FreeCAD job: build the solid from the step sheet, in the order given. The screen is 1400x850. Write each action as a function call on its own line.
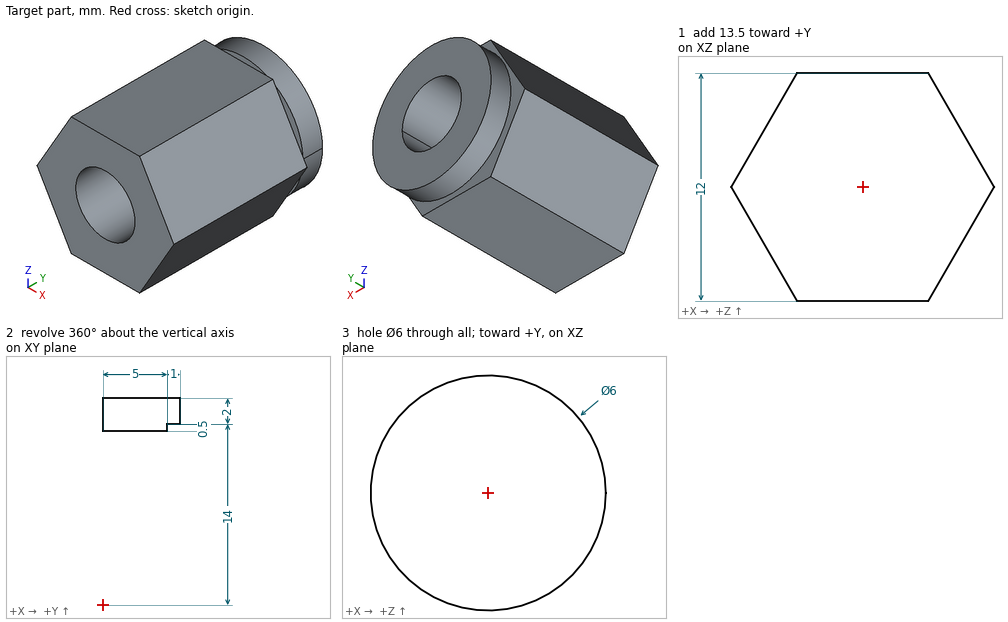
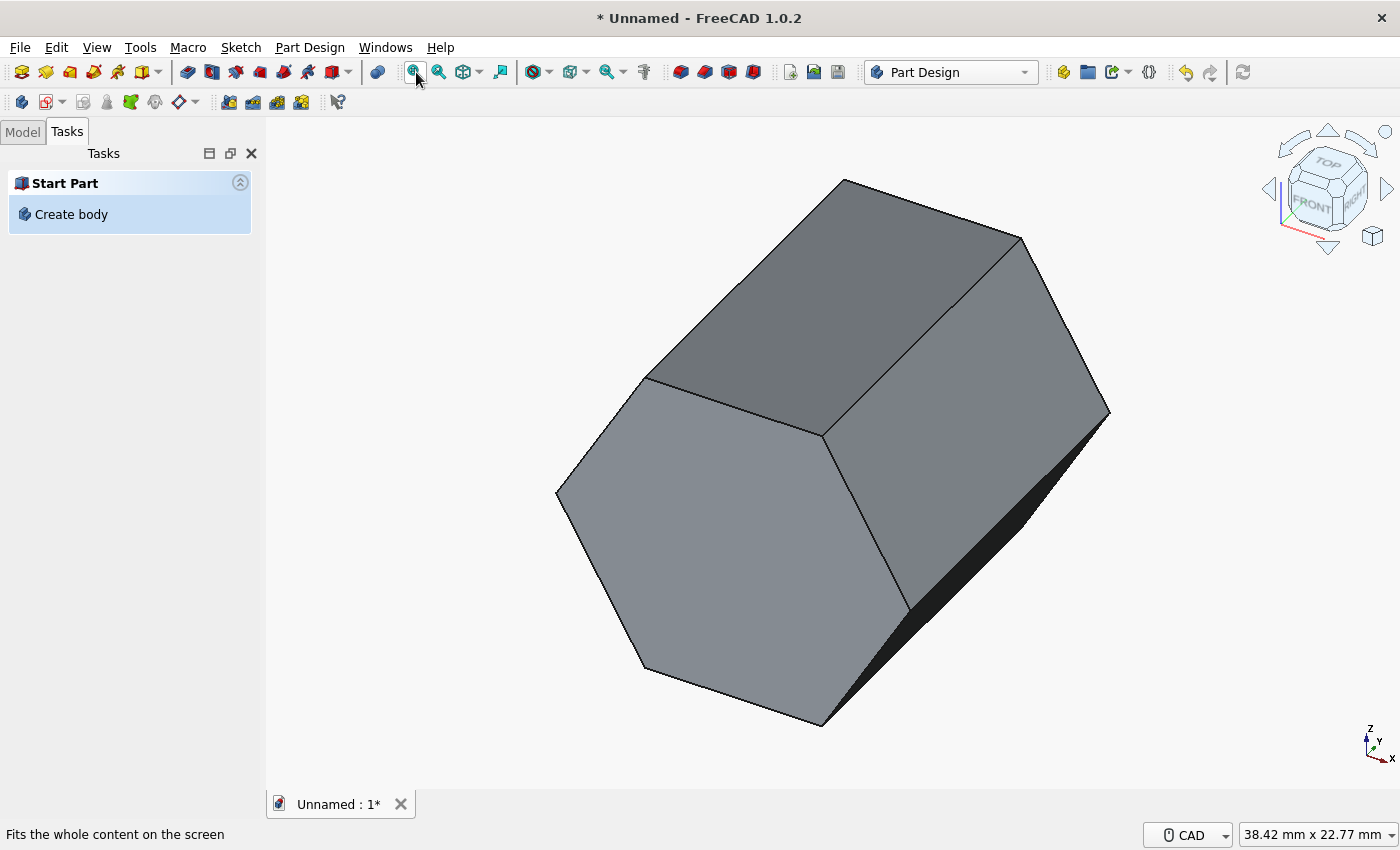
click(46, 102)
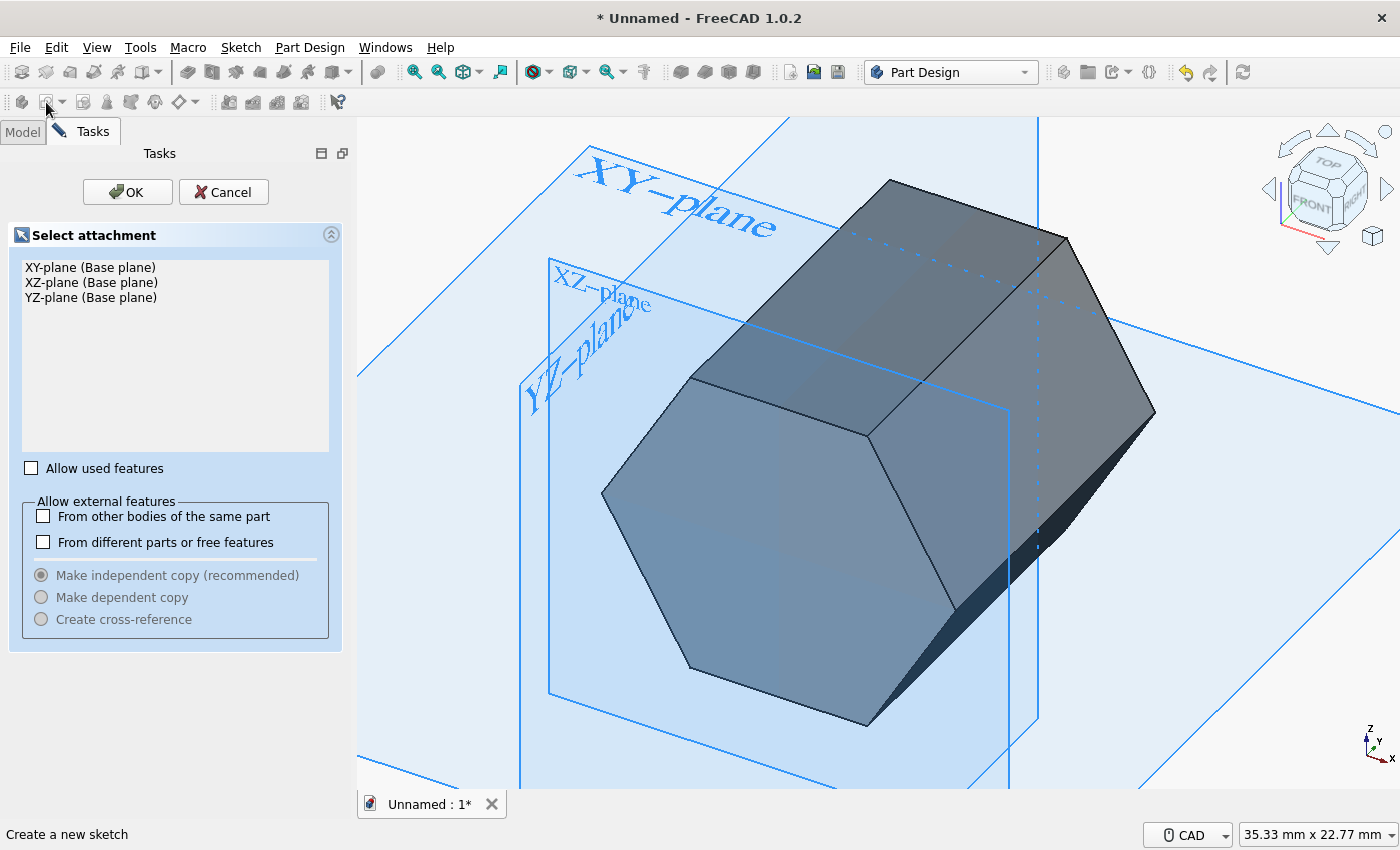
click(82, 268)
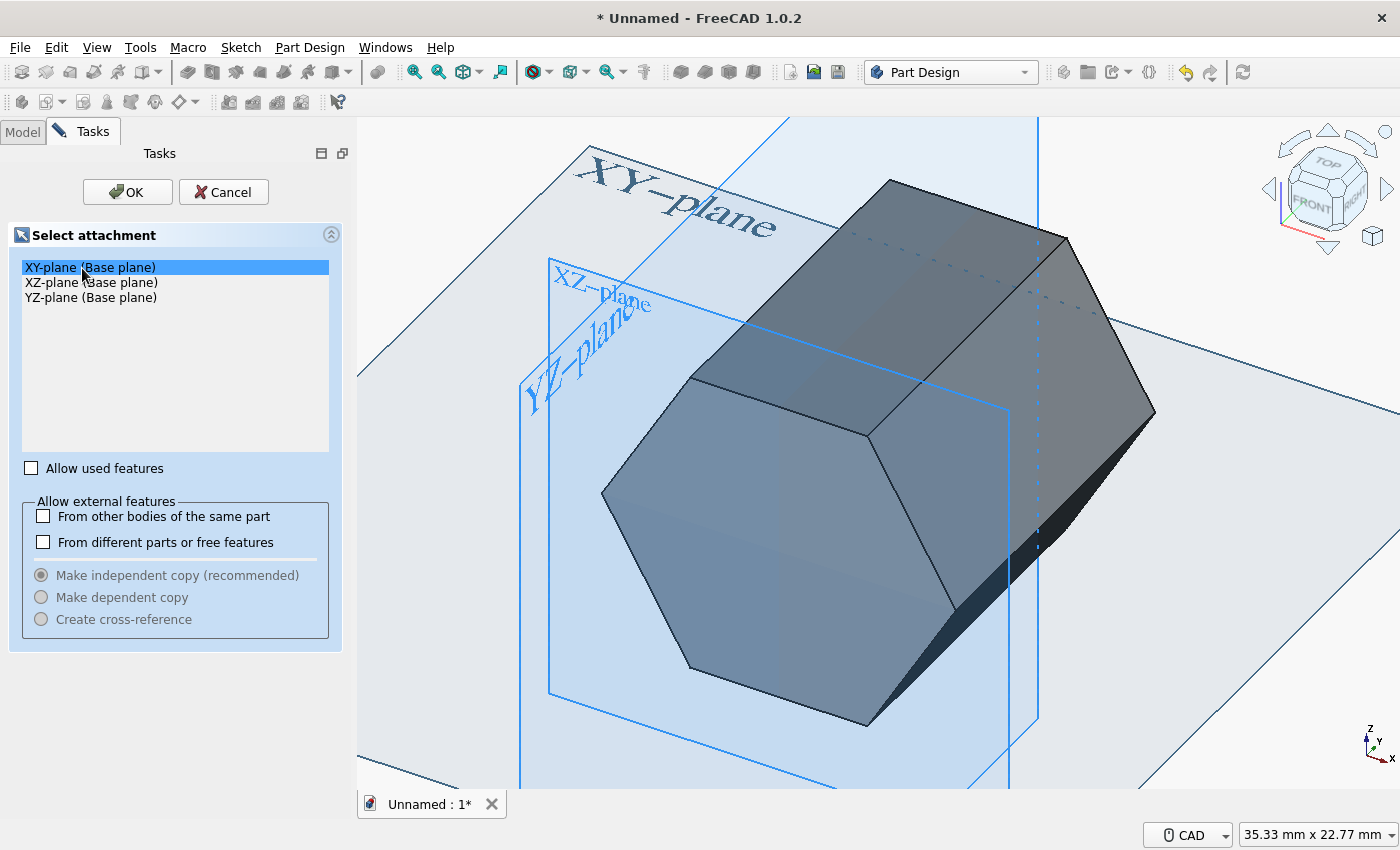
click(128, 192)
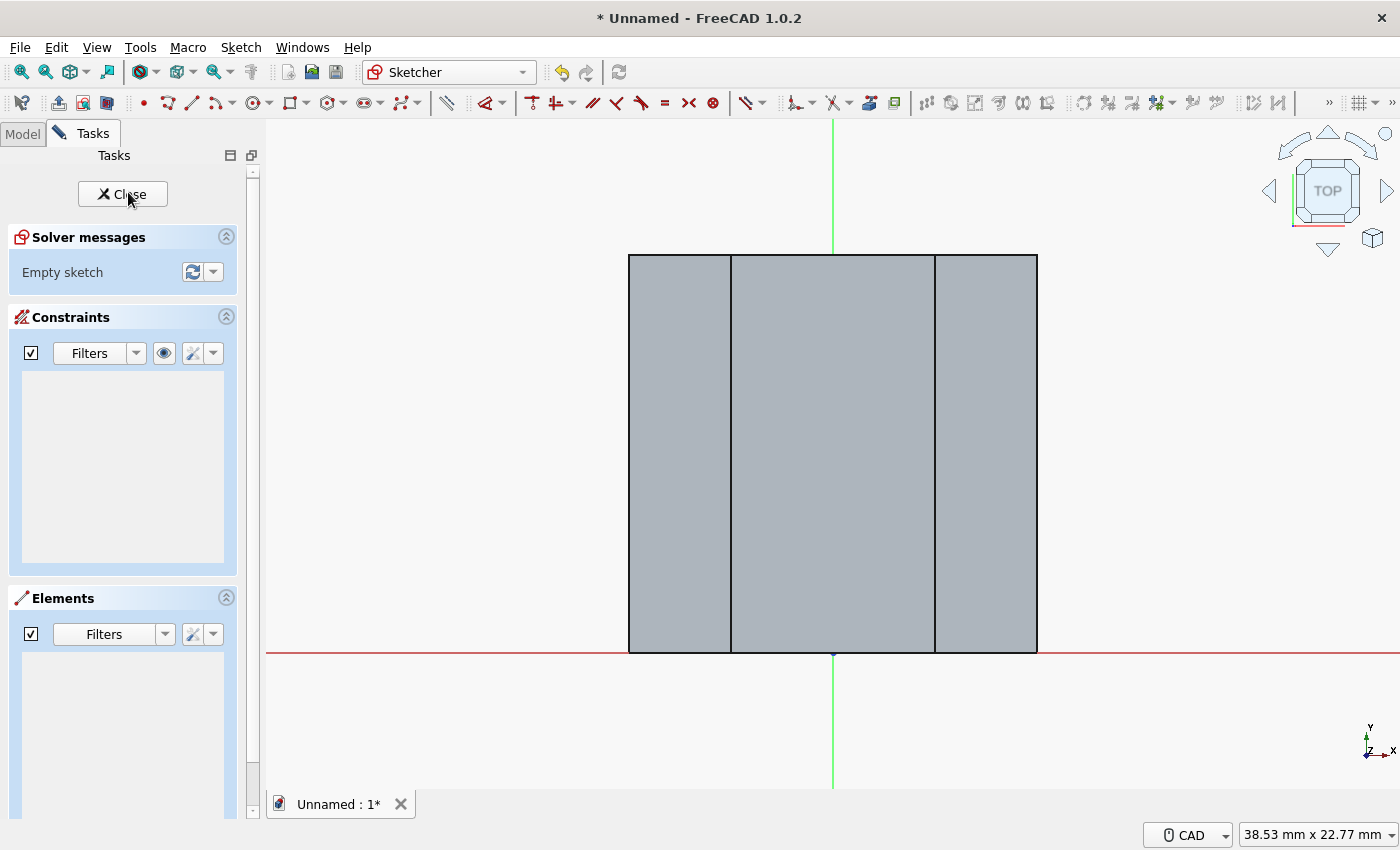
click(108, 104)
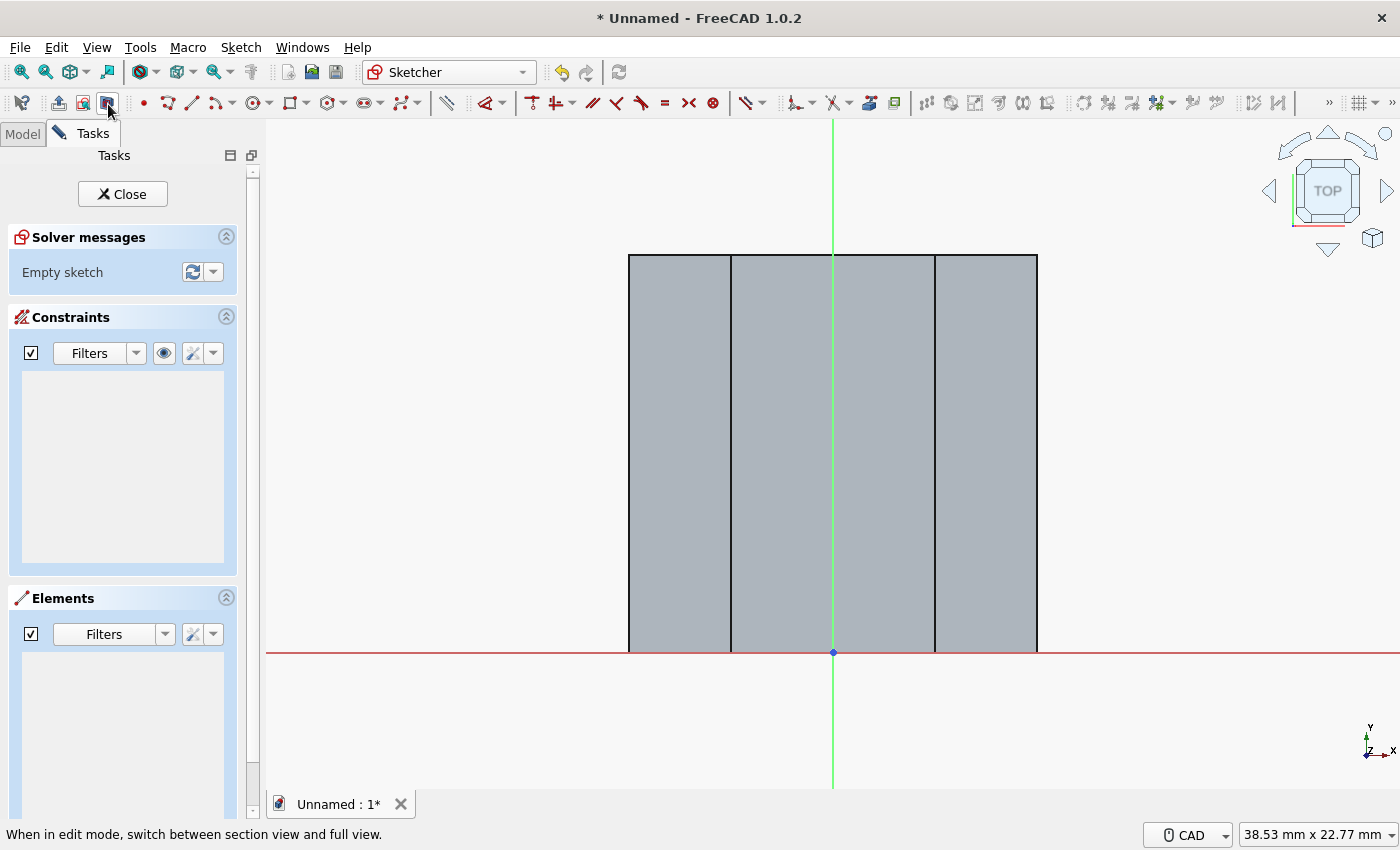
scroll(973, 147, up, 7)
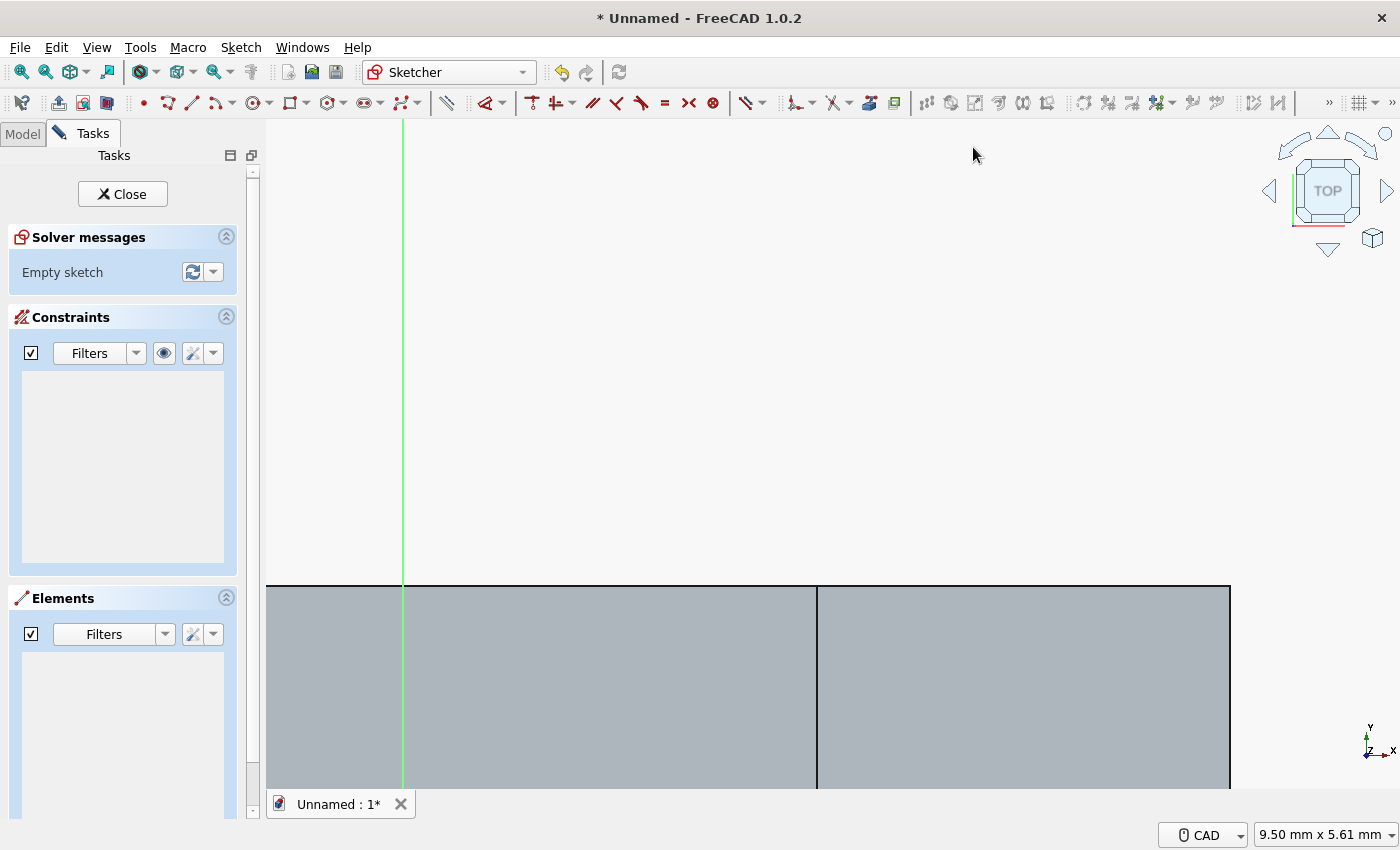
click(168, 104)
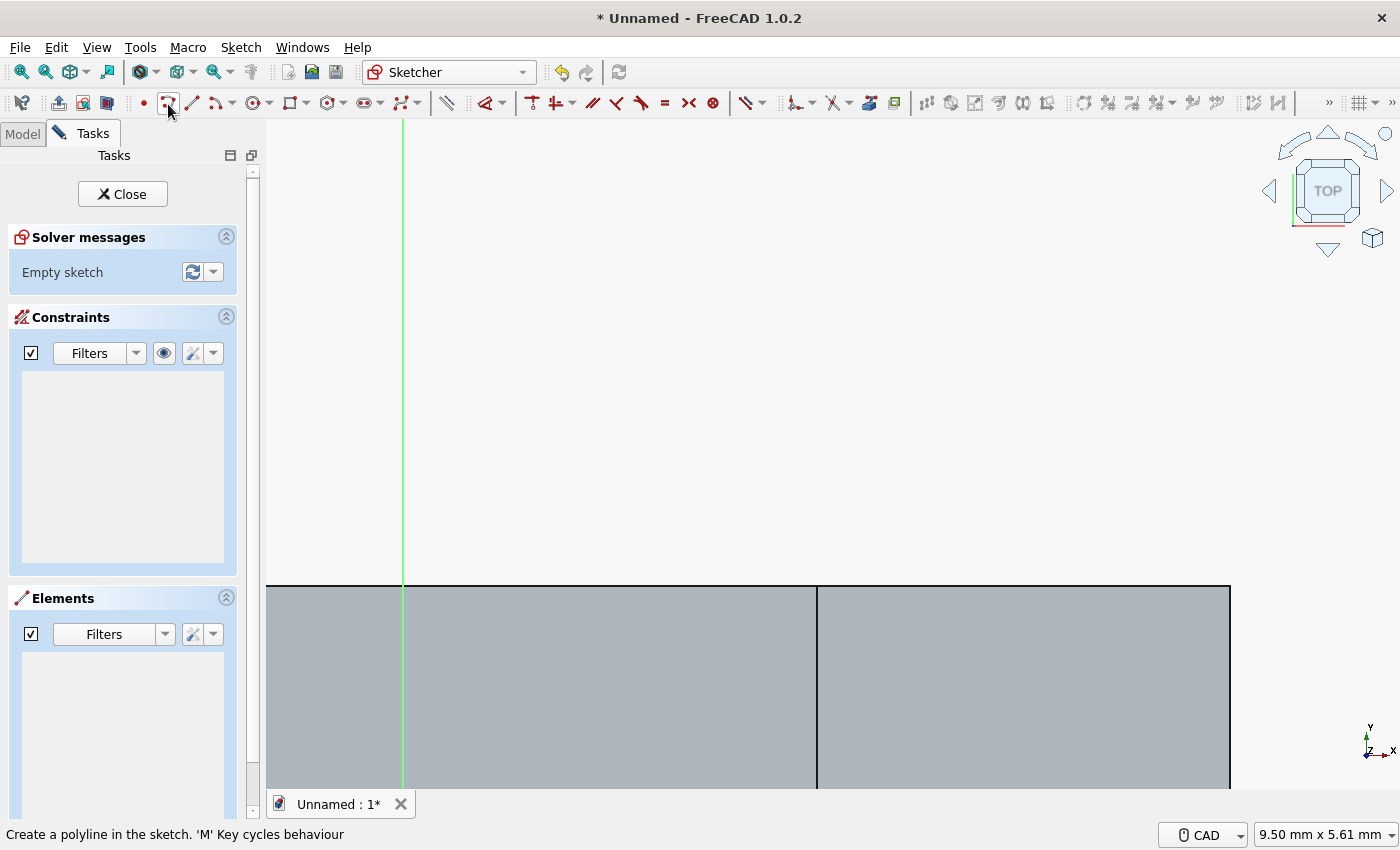
click(403, 586)
click(1000, 586)
click(1000, 527)
click(1119, 527)
click(1119, 288)
click(412, 288)
click(403, 587)
key(Escape)
key(Escape)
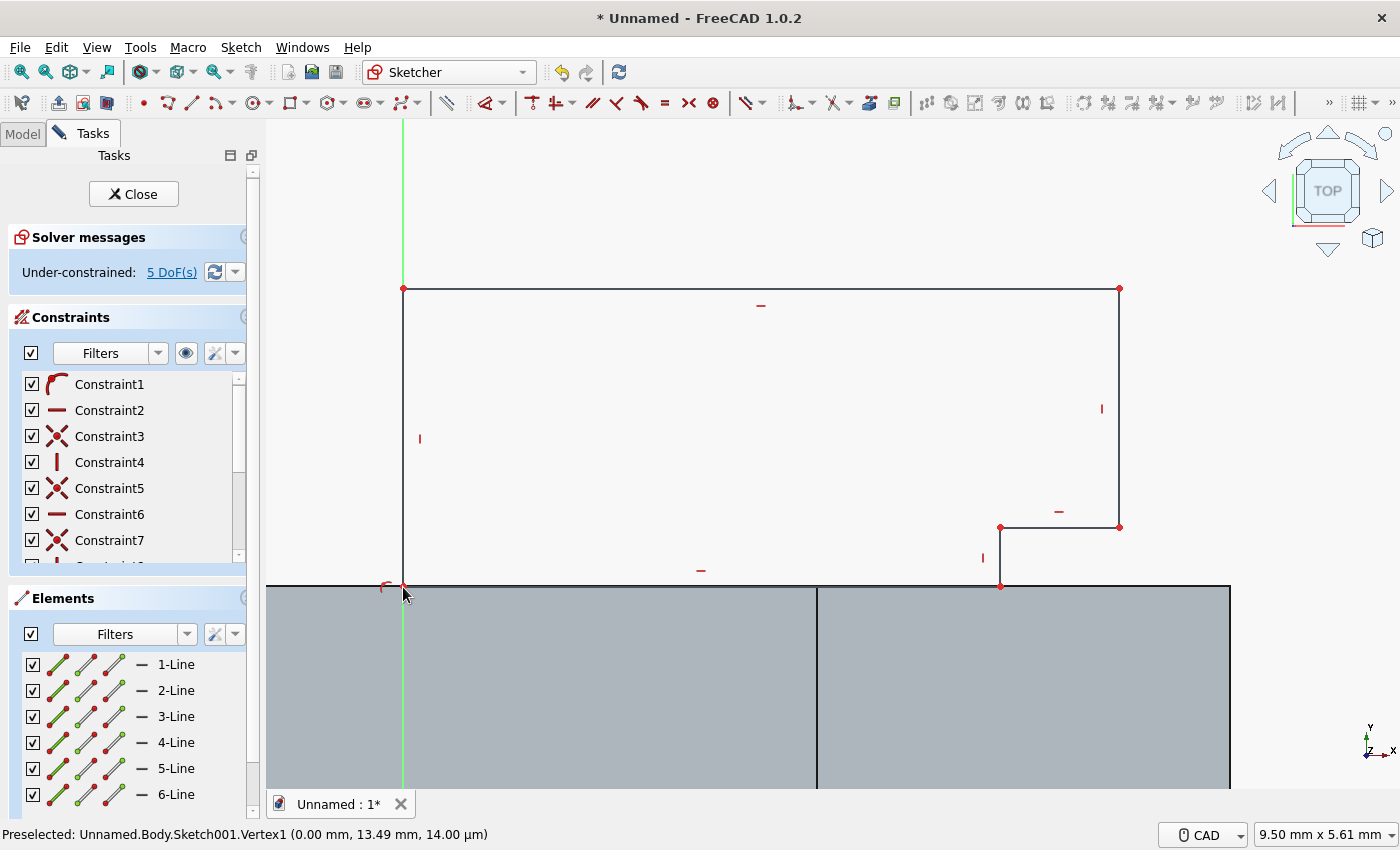
click(486, 104)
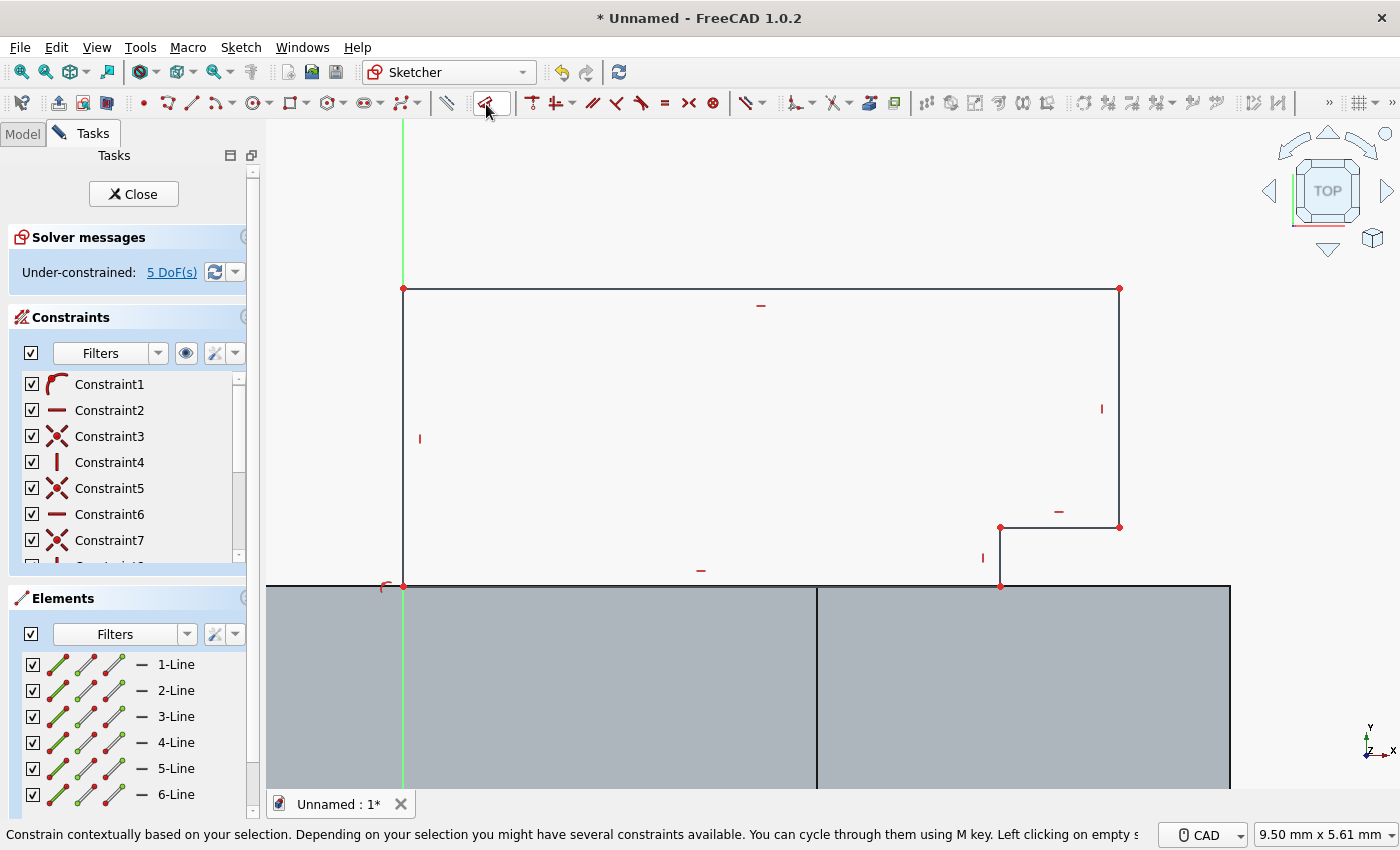
click(582, 587)
click(702, 621)